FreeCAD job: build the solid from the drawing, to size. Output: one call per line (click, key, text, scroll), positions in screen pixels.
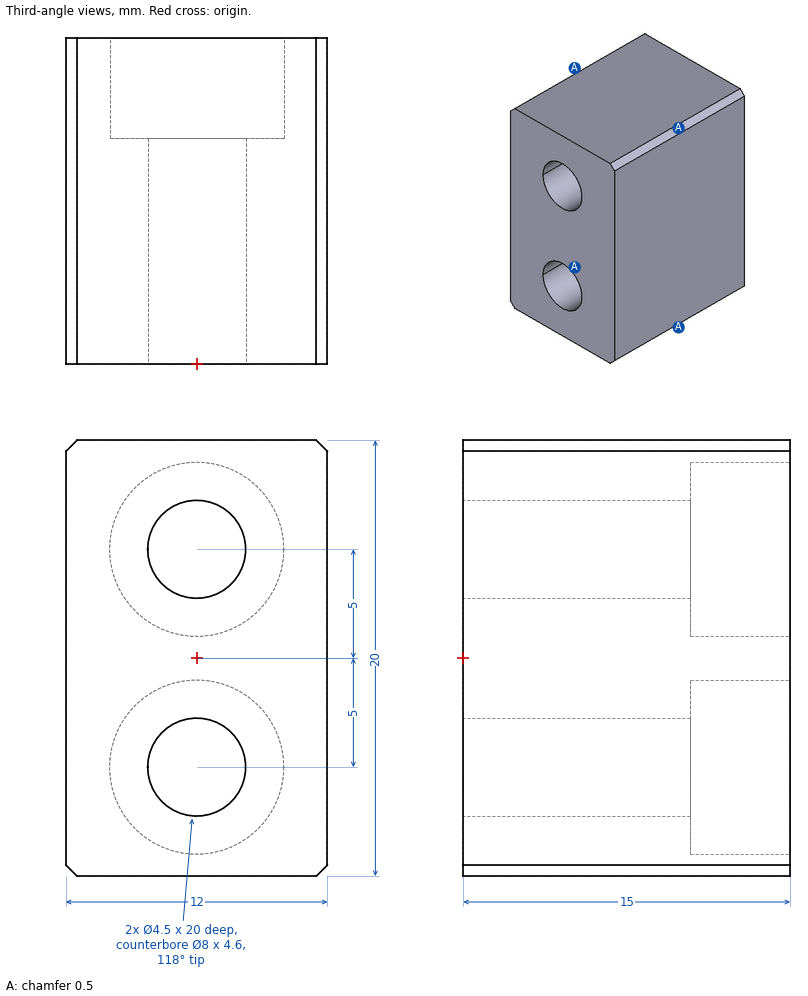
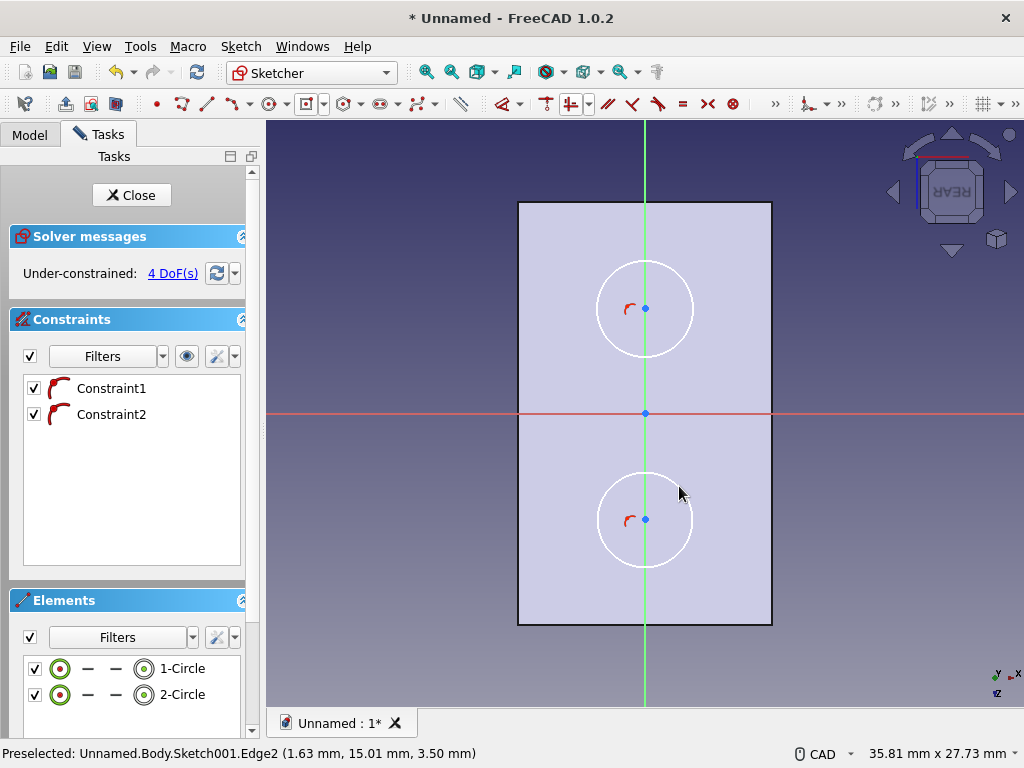
click(679, 275)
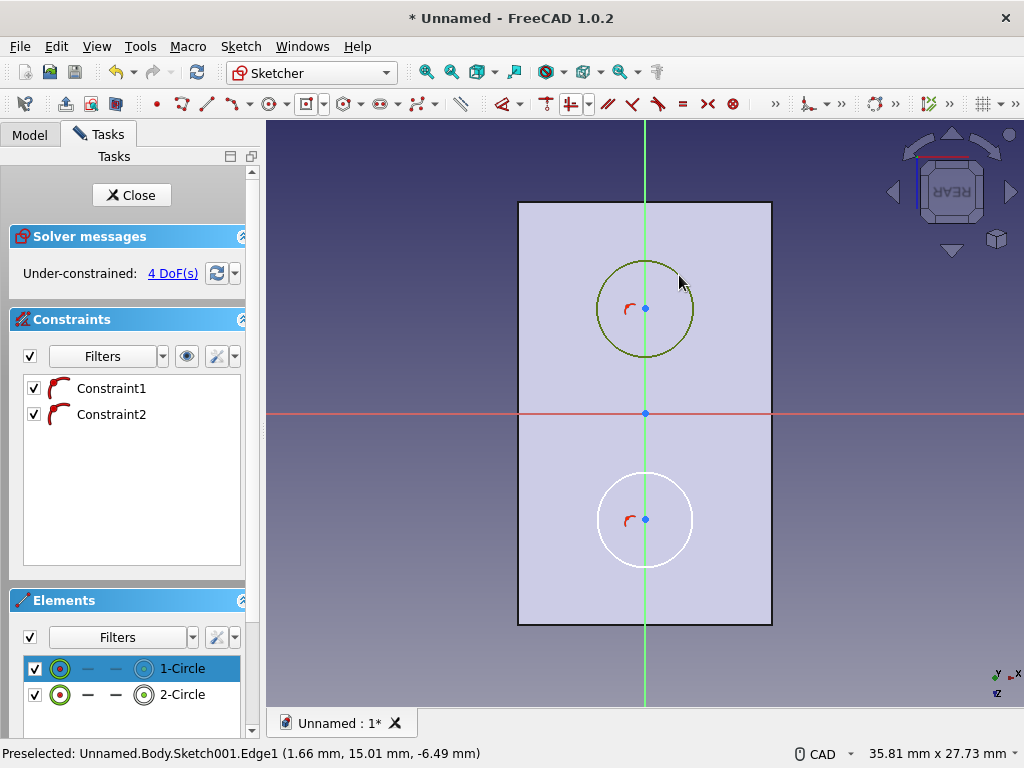
click(678, 486)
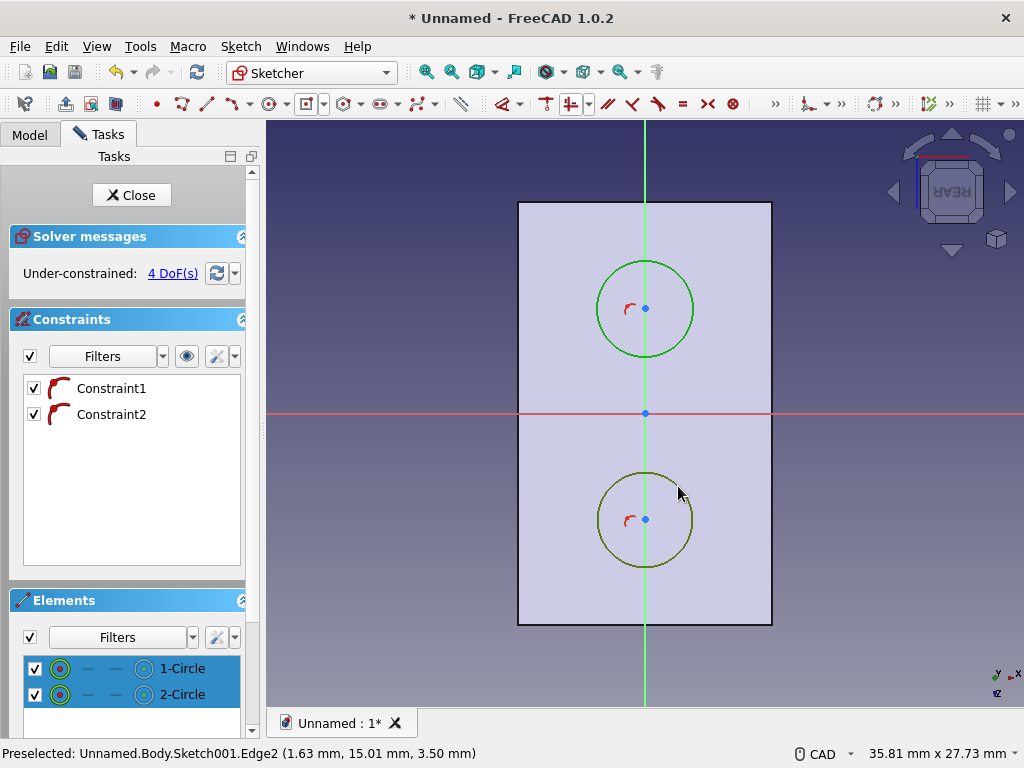
click(683, 104)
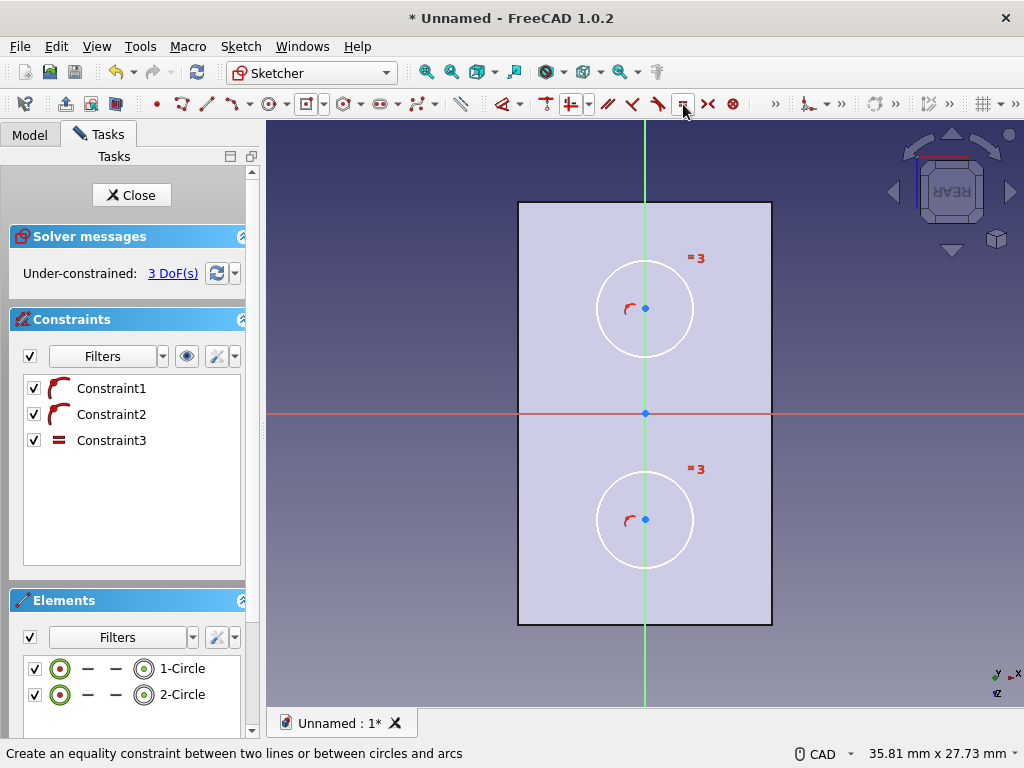
click(679, 275)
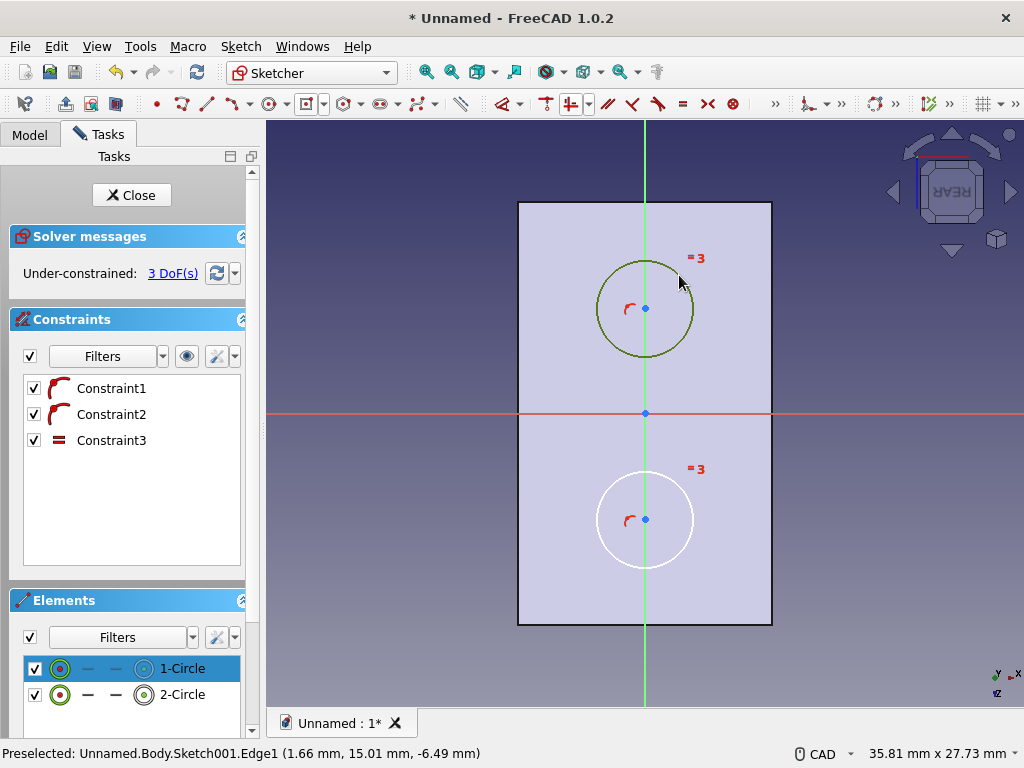
key(k)
key(o)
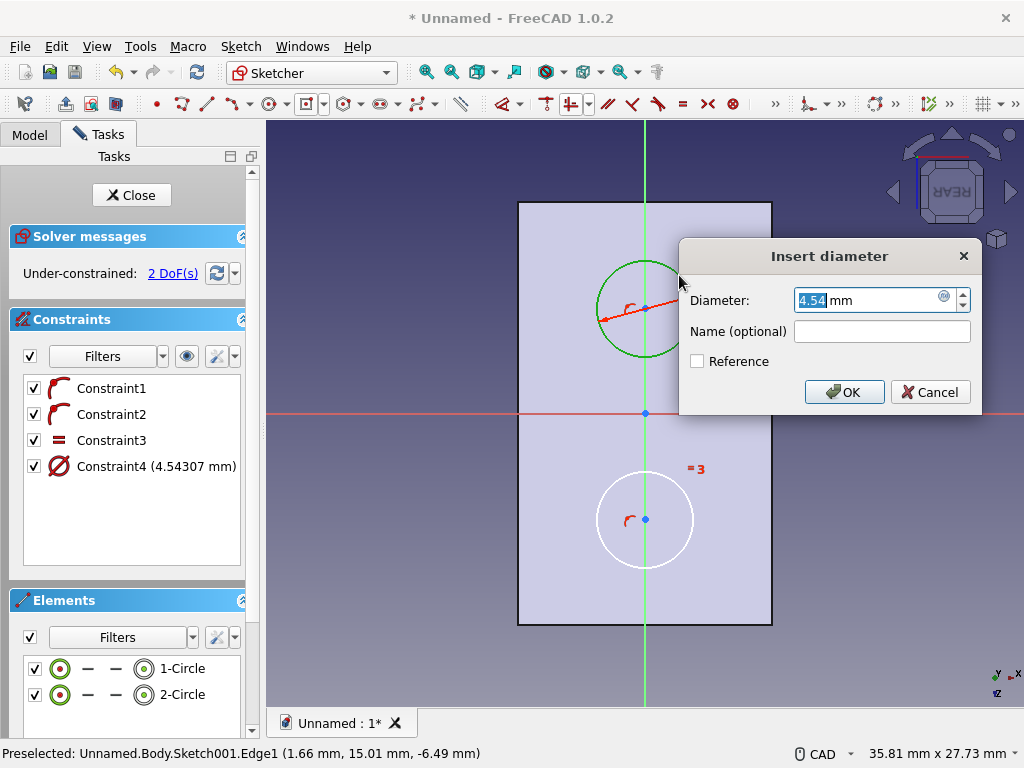
text(4.5)
key(Return)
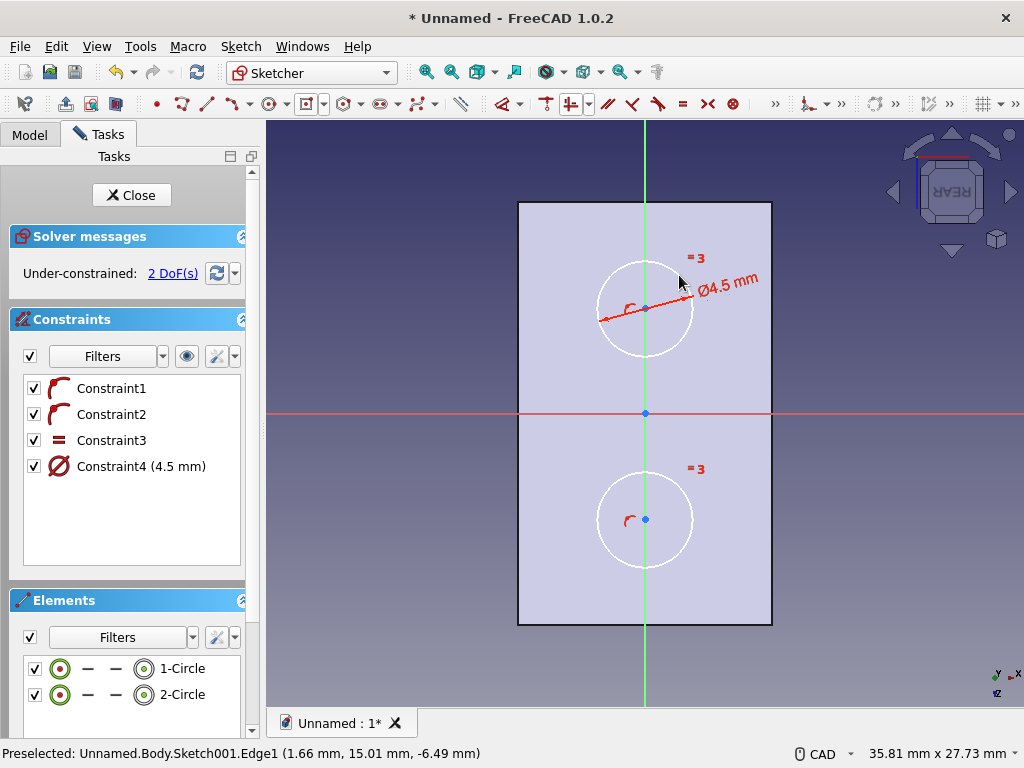
click(645, 309)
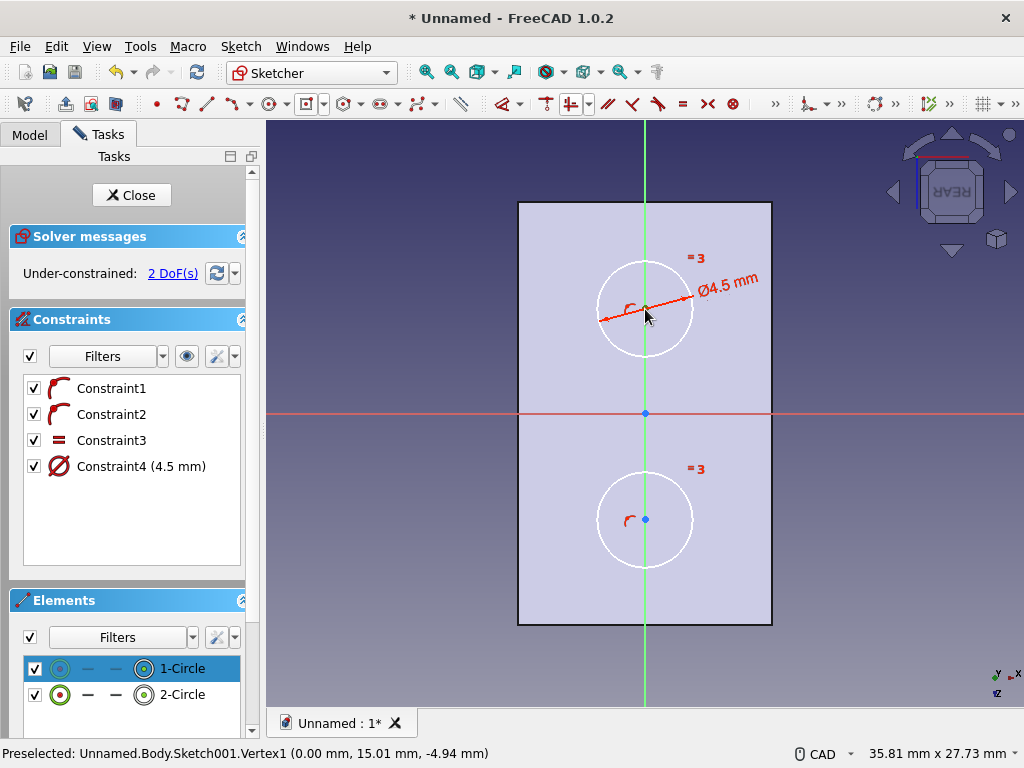
click(520, 104)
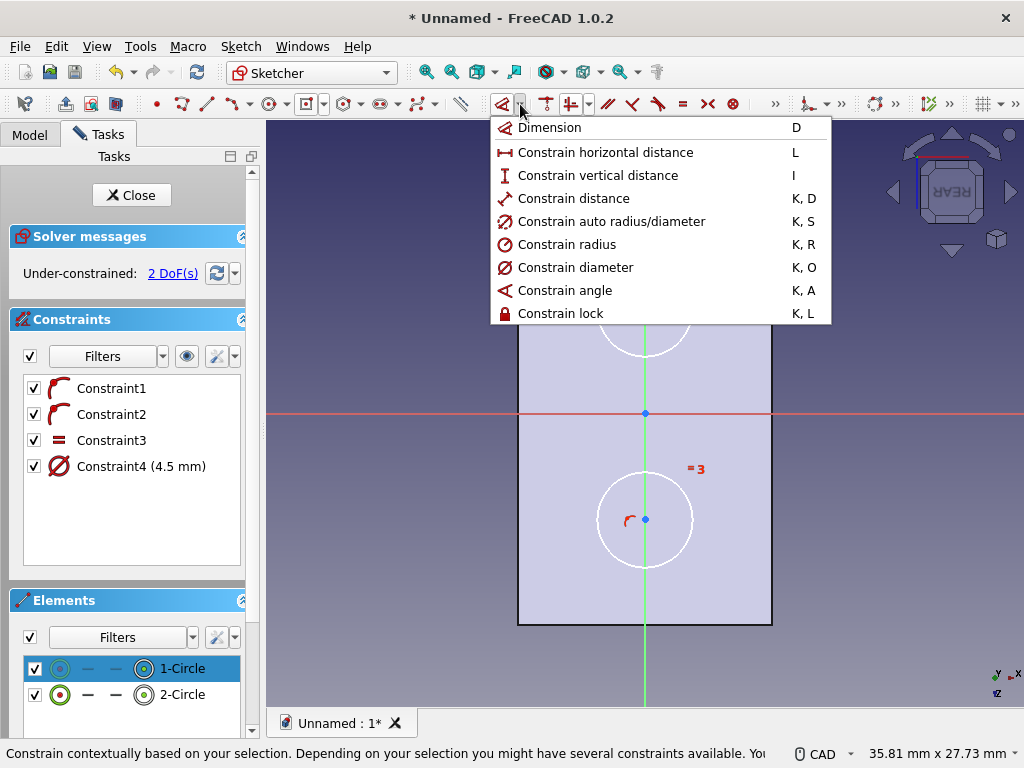
click(661, 176)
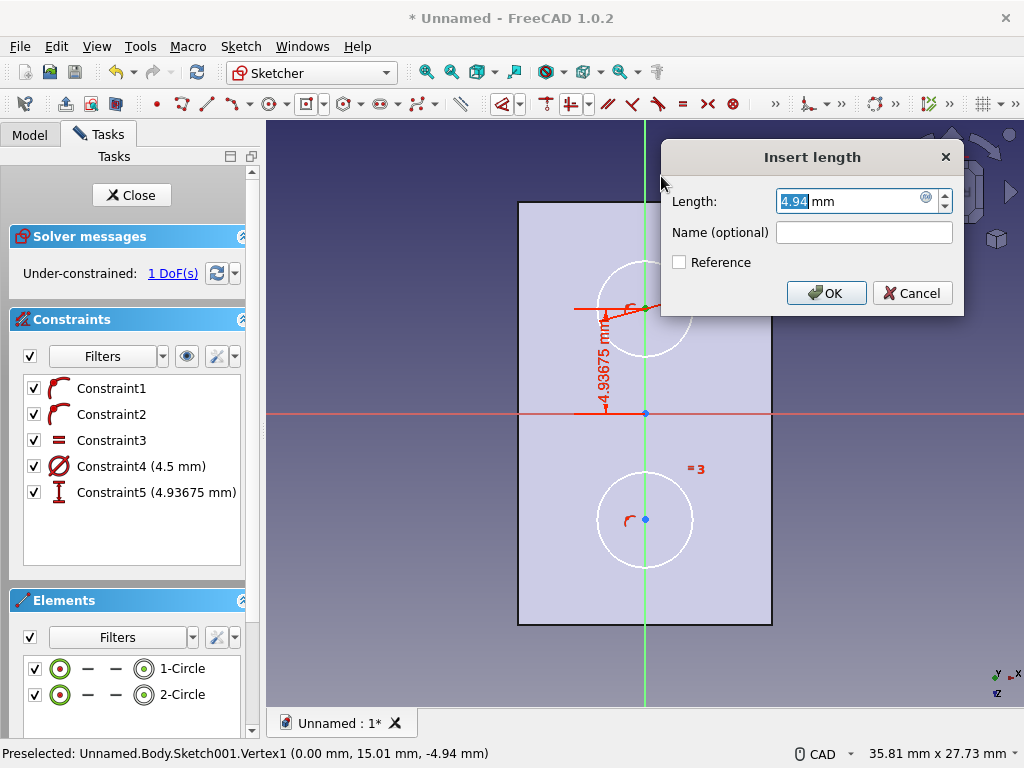
text(5)
key(Return)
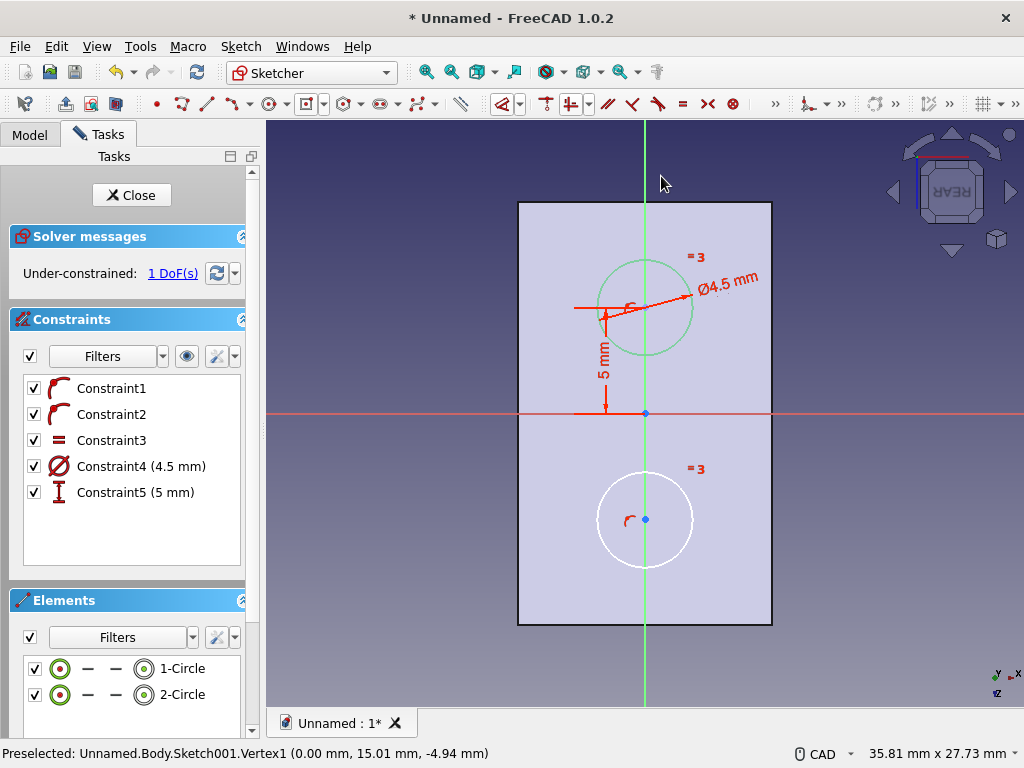
click(645, 520)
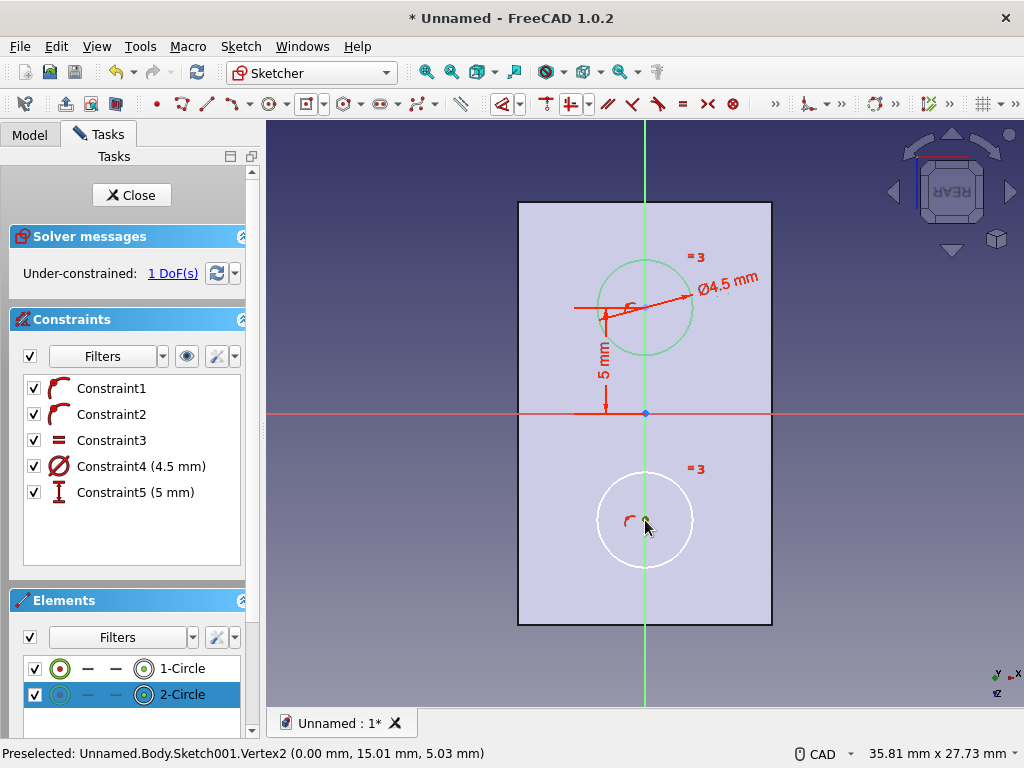
key(i)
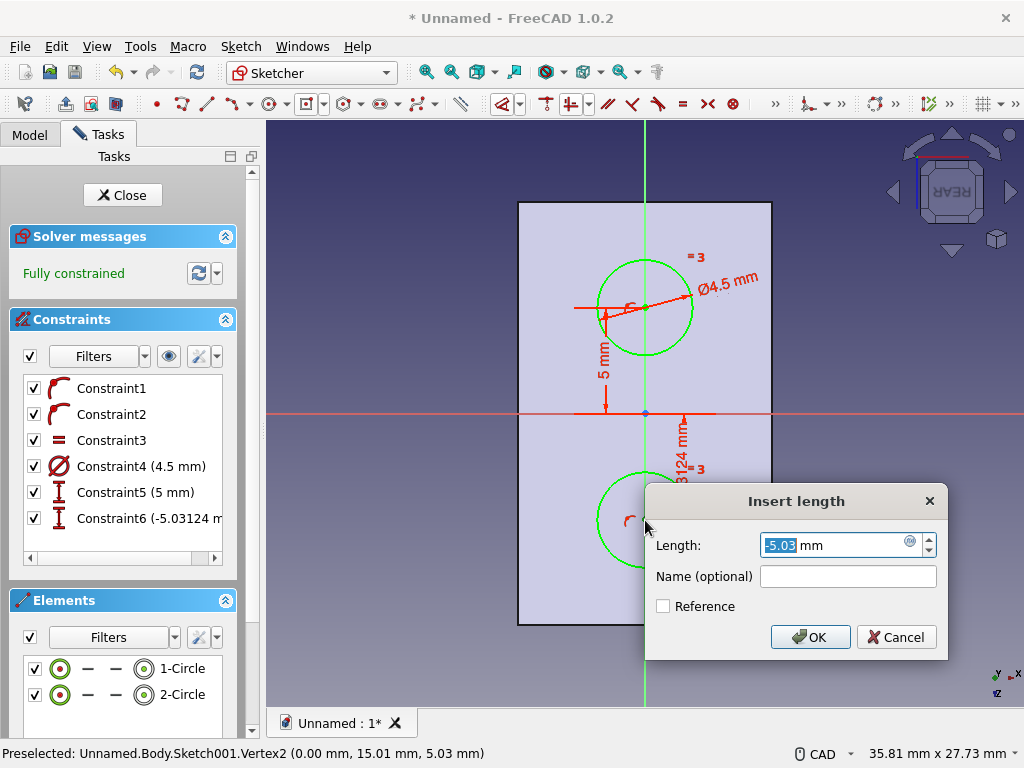
text(-5)
key(Return)